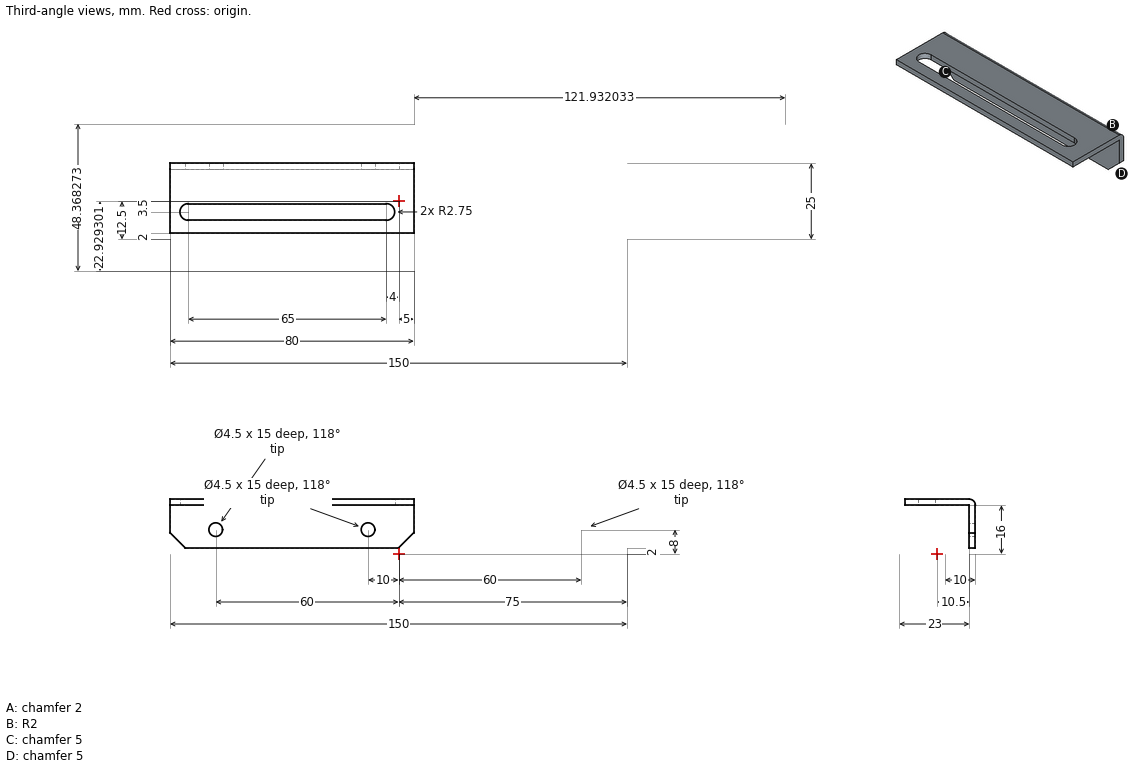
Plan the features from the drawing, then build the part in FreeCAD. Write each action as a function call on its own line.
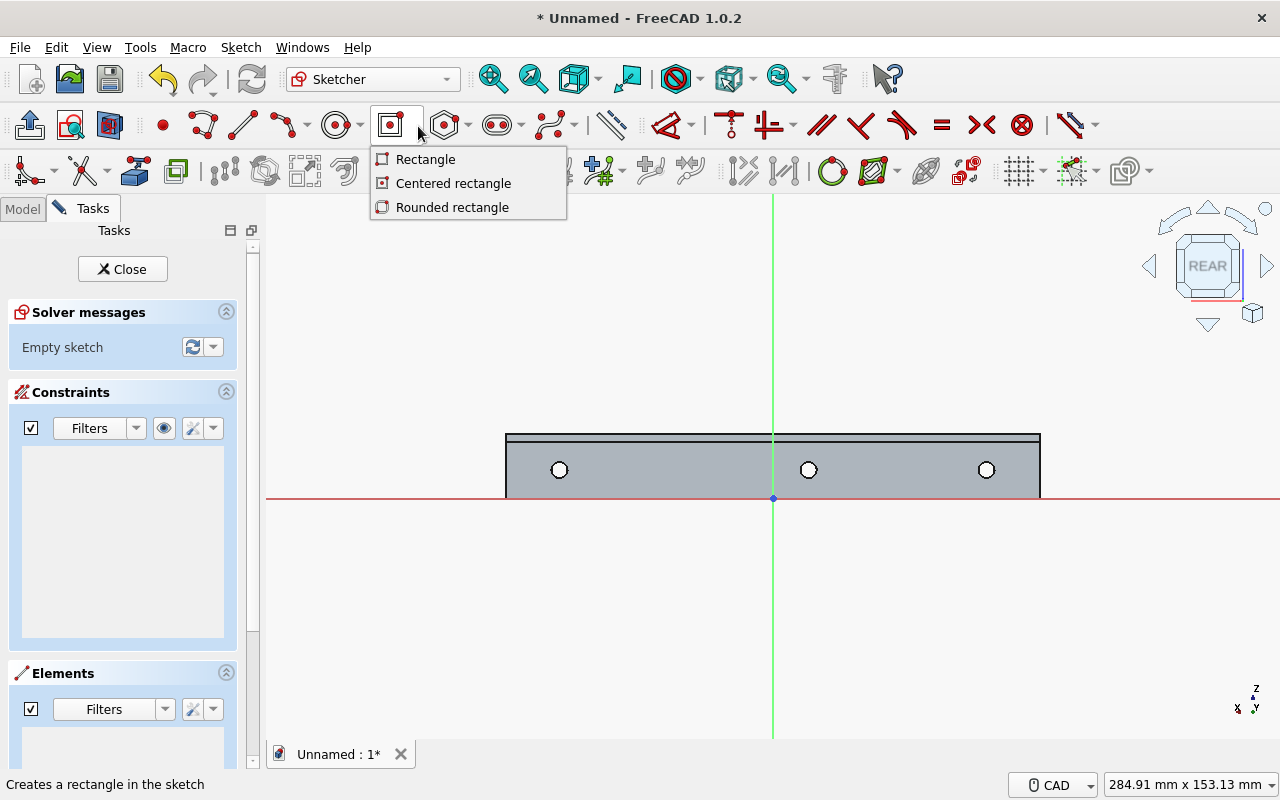
click(468, 159)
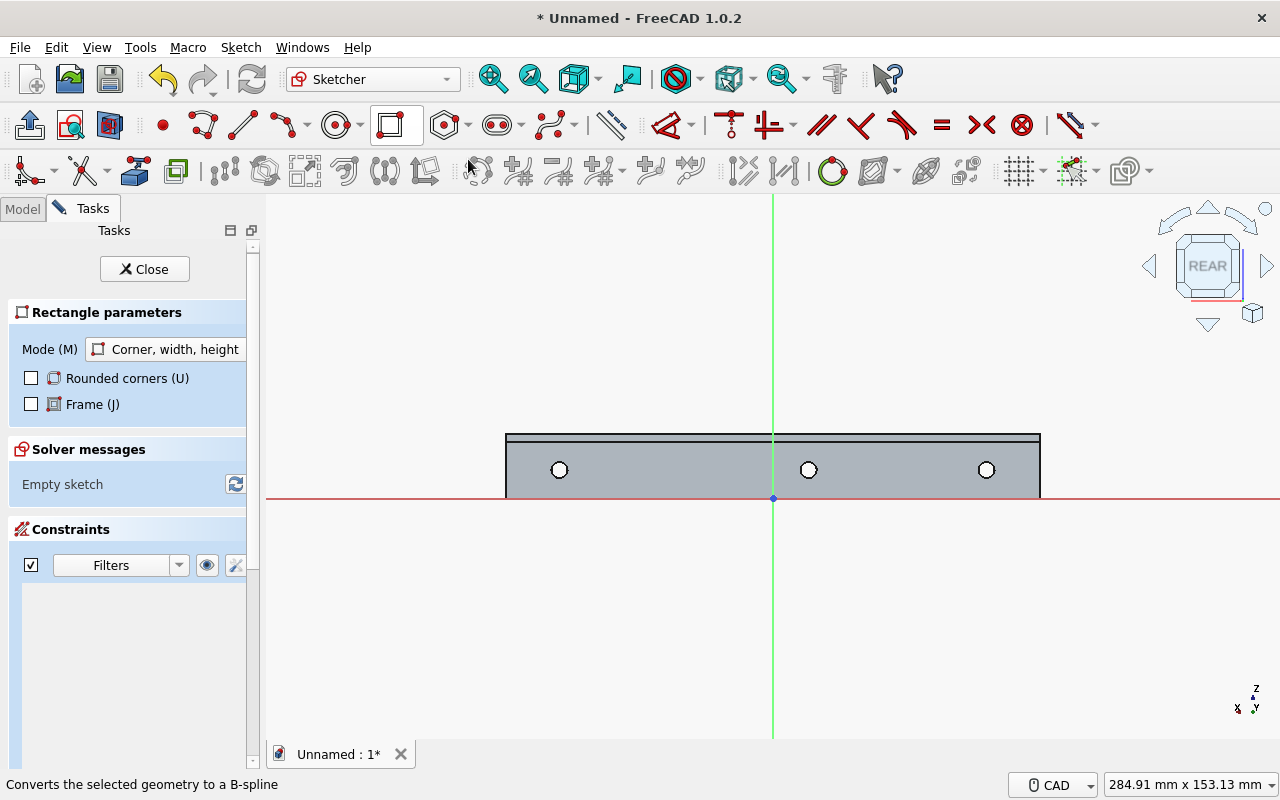
scroll(506, 491, up, 5)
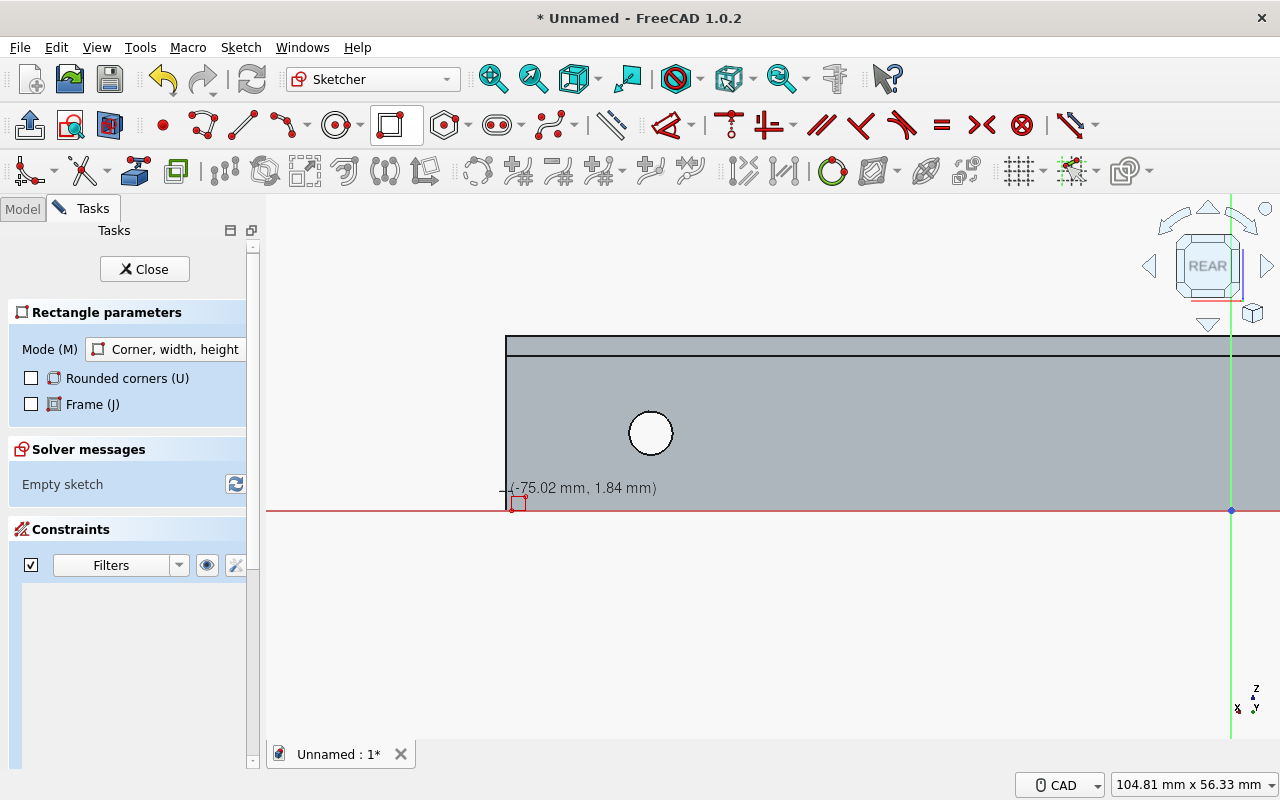
click(506, 491)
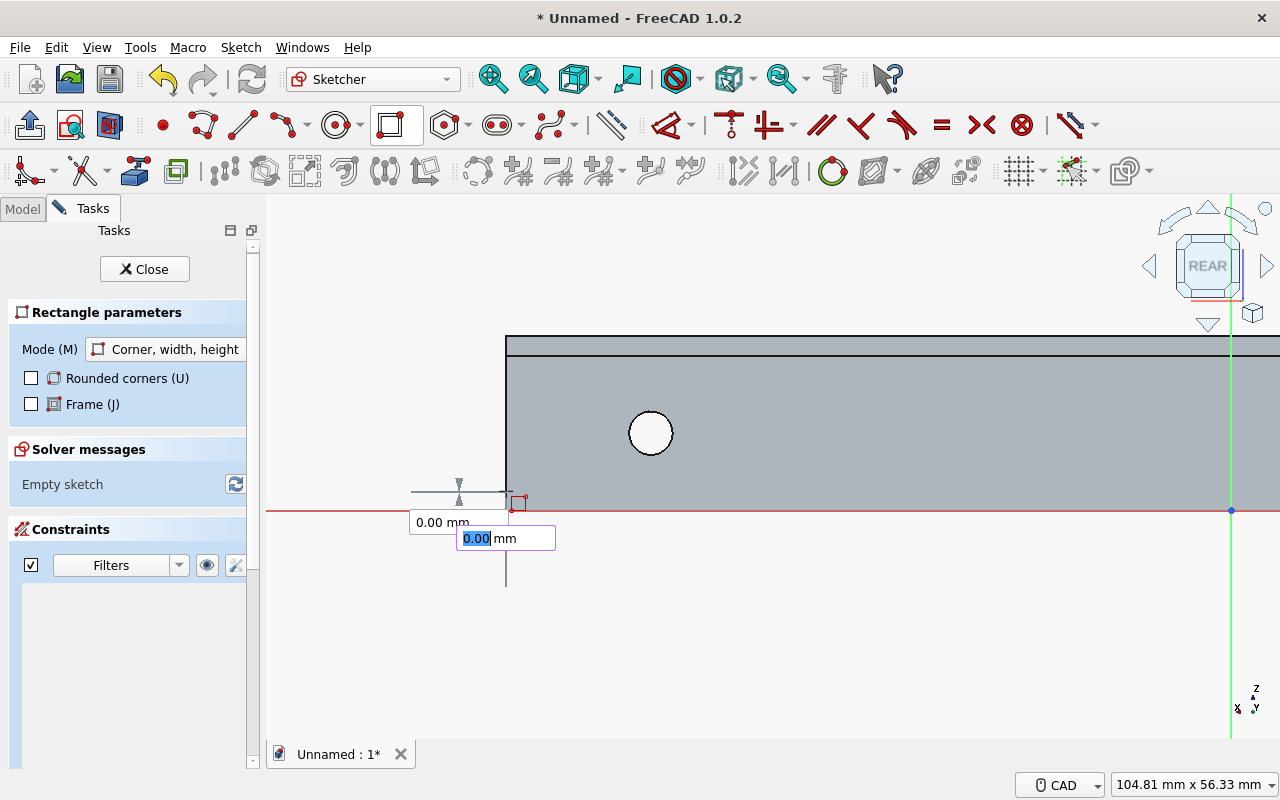
scroll(398, 447, down, 5)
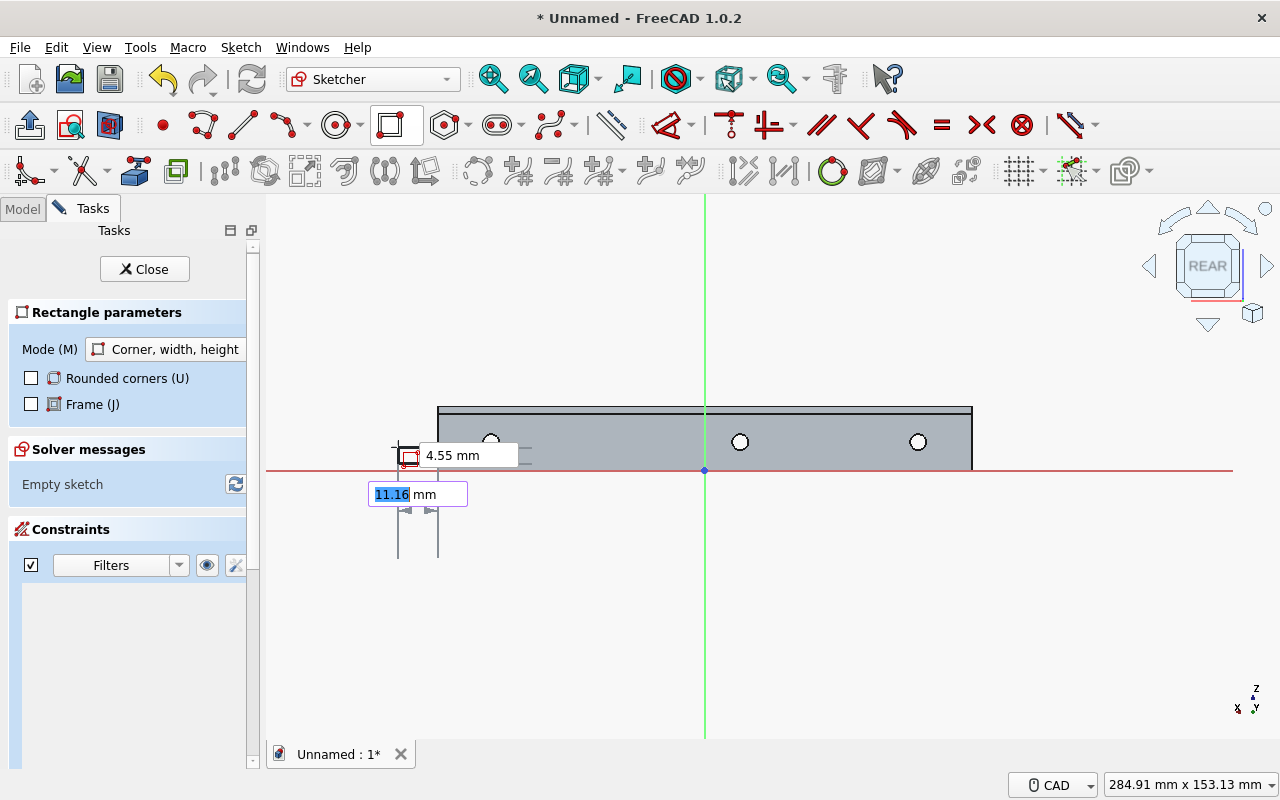
click(972, 471)
key(Escape)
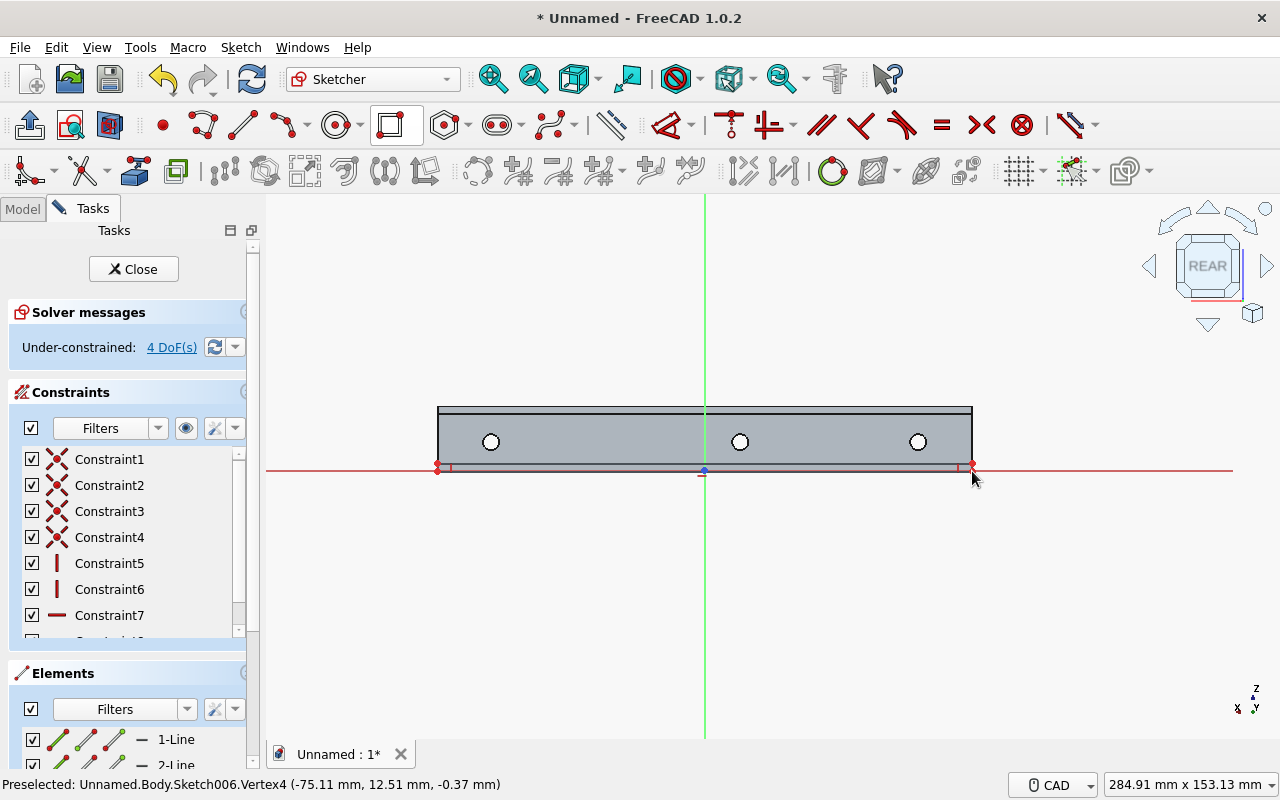
scroll(438, 472, up, 3)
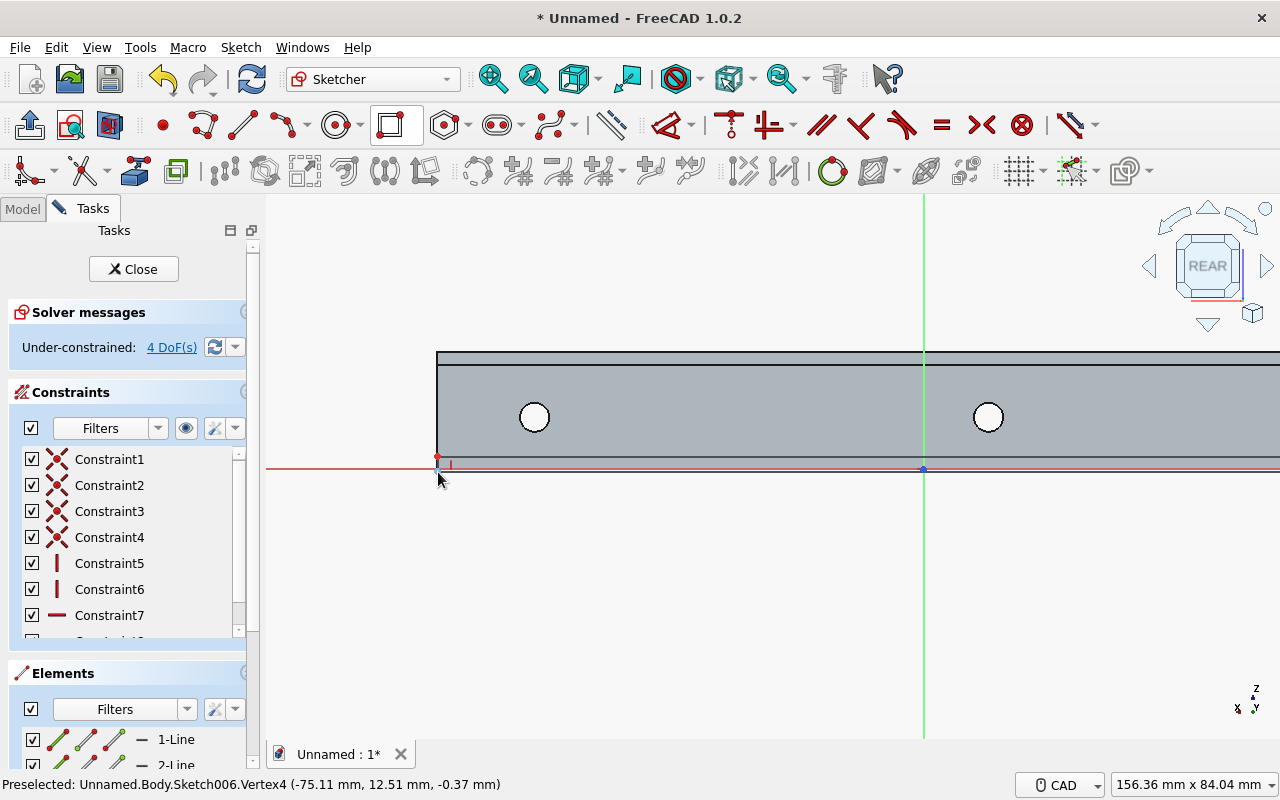
click(438, 472)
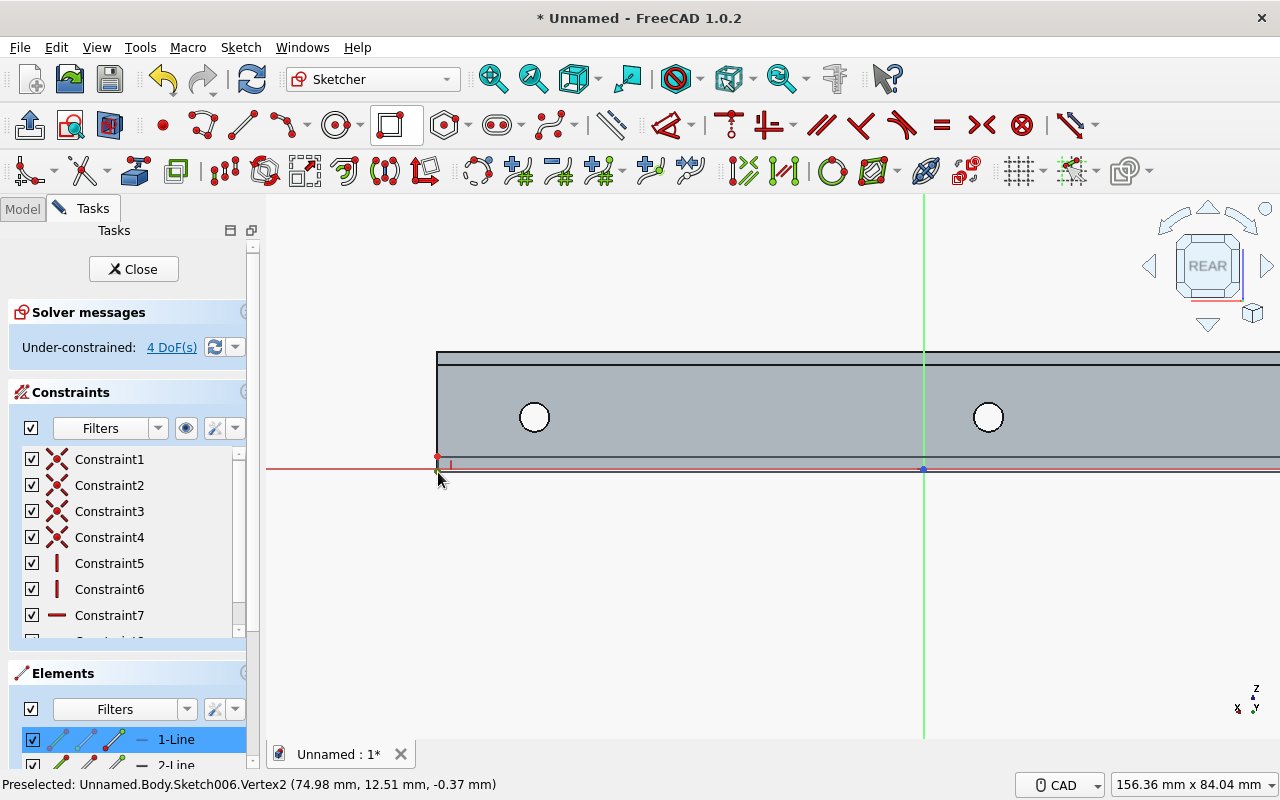
click(353, 469)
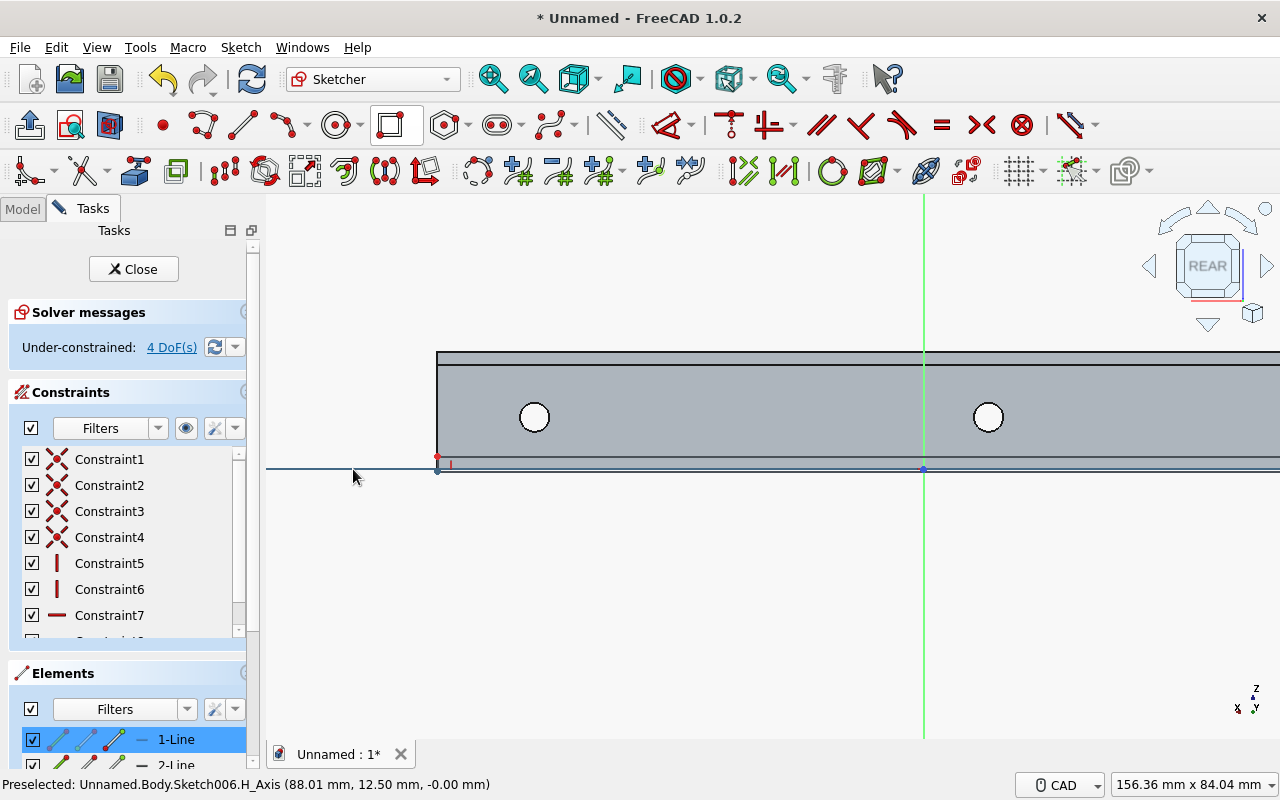
key(c)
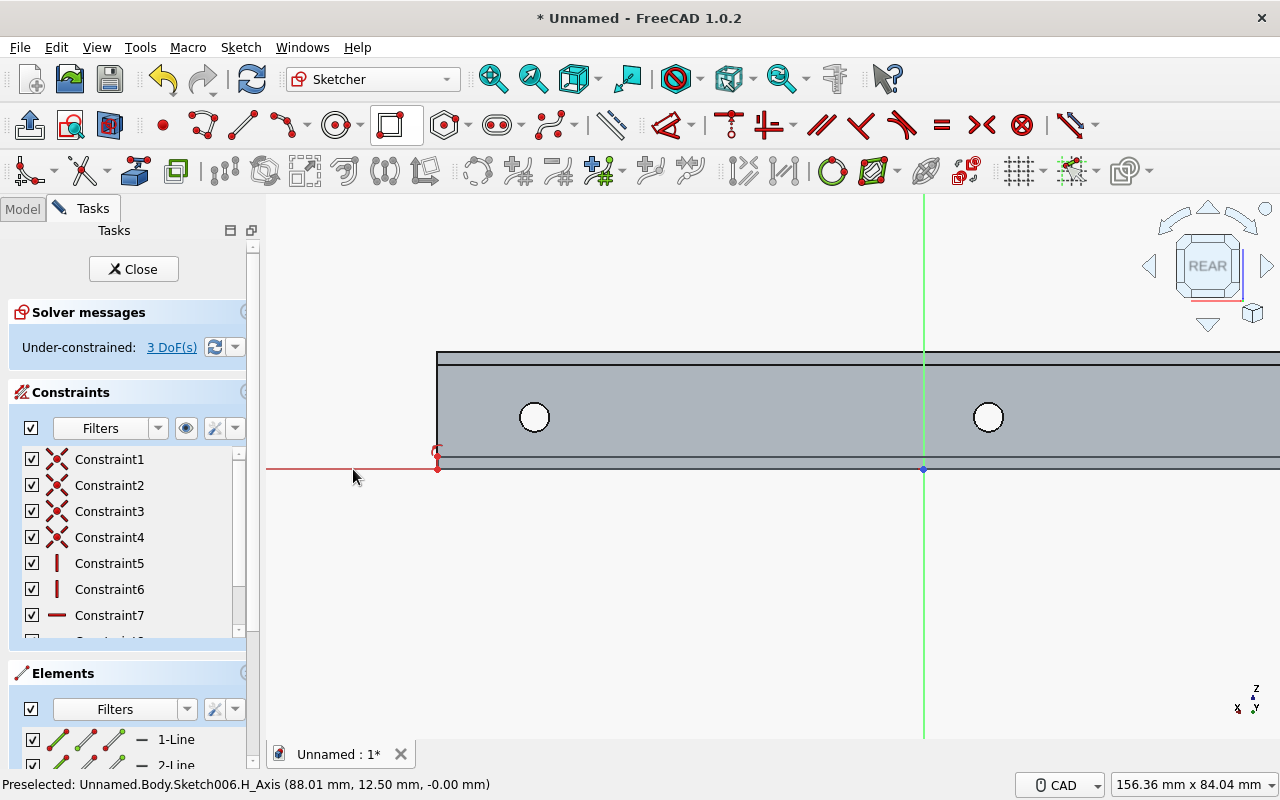
click(666, 126)